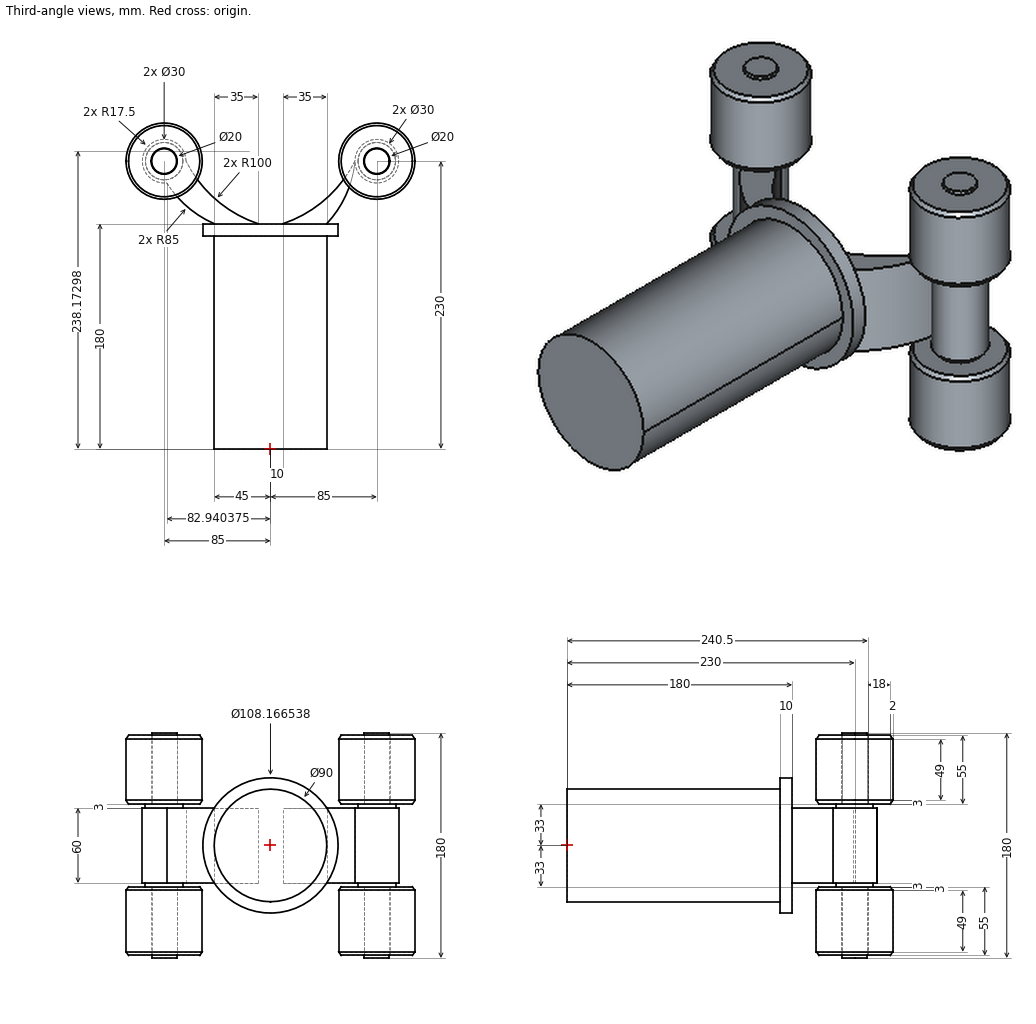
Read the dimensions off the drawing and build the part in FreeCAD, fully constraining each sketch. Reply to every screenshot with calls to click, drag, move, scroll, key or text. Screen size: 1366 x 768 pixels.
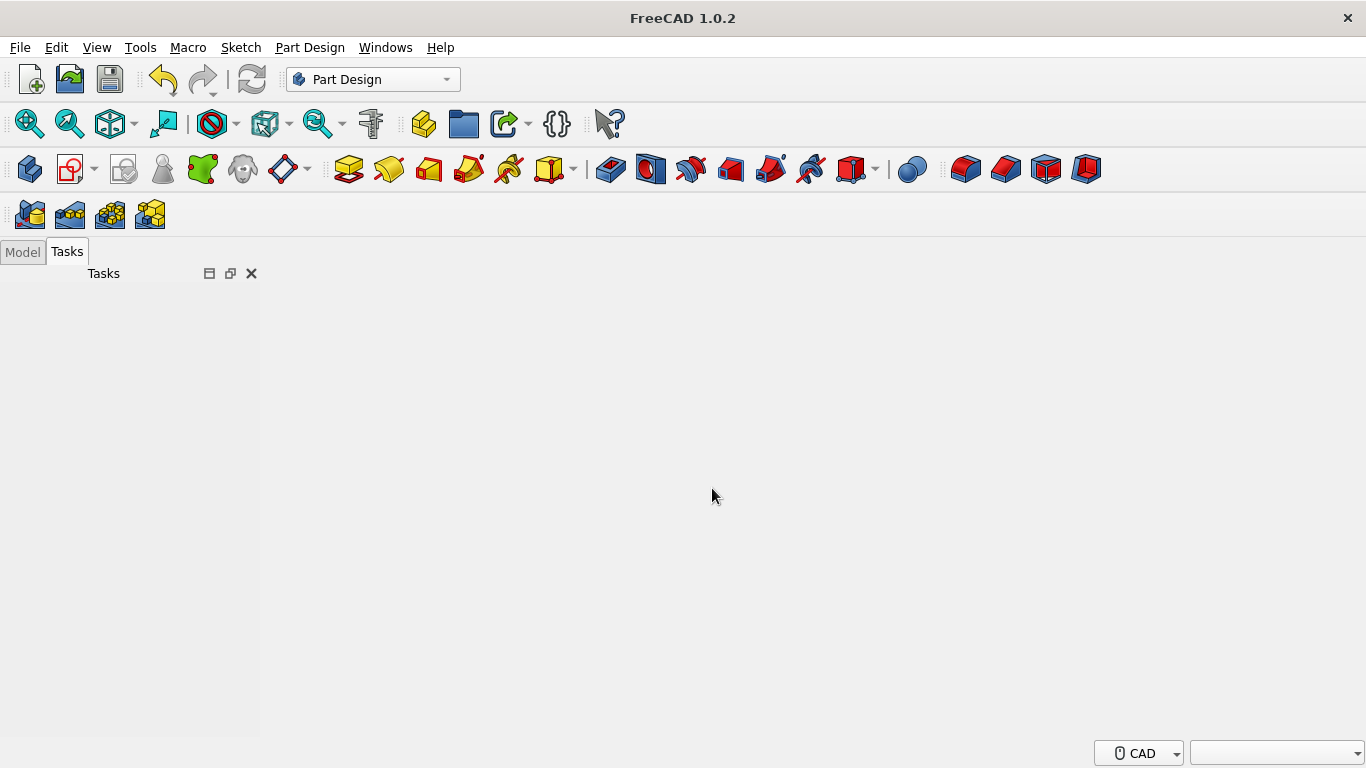
click(30, 80)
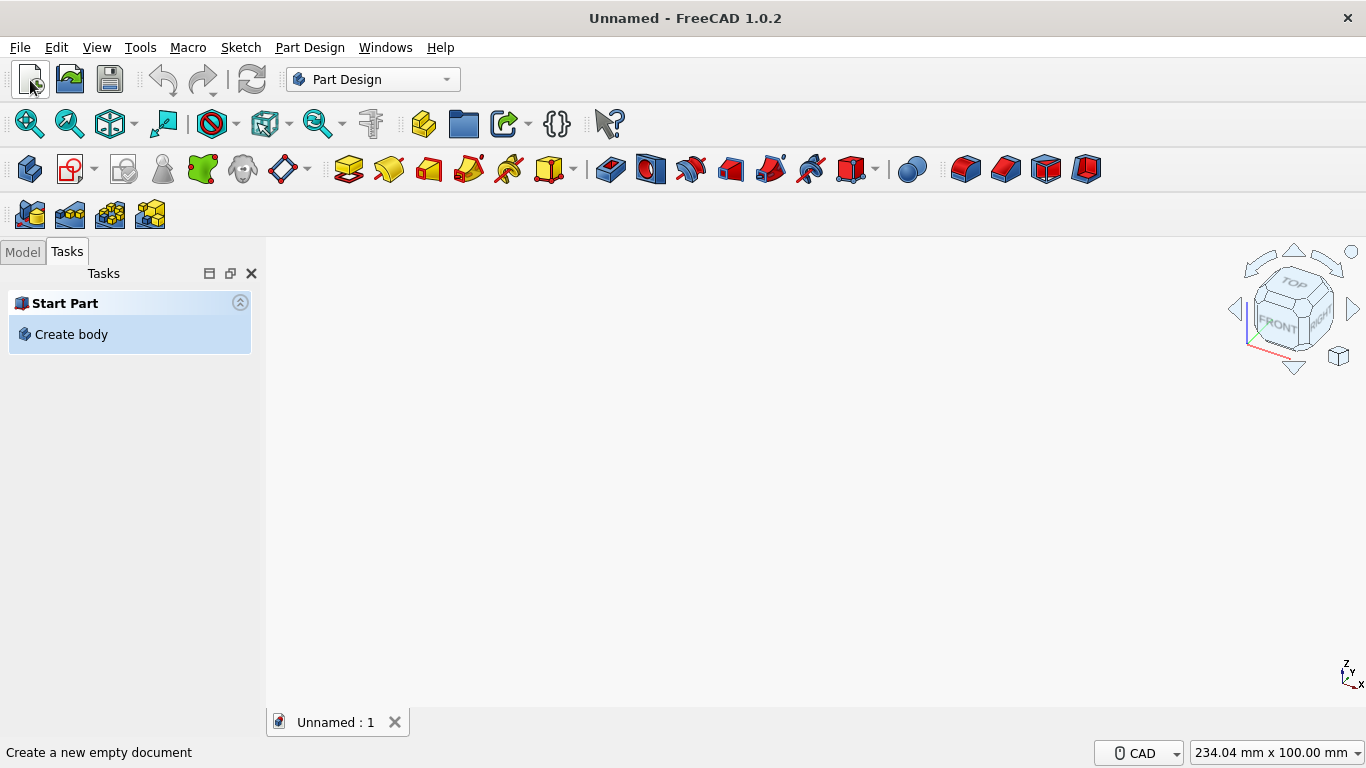
click(70, 170)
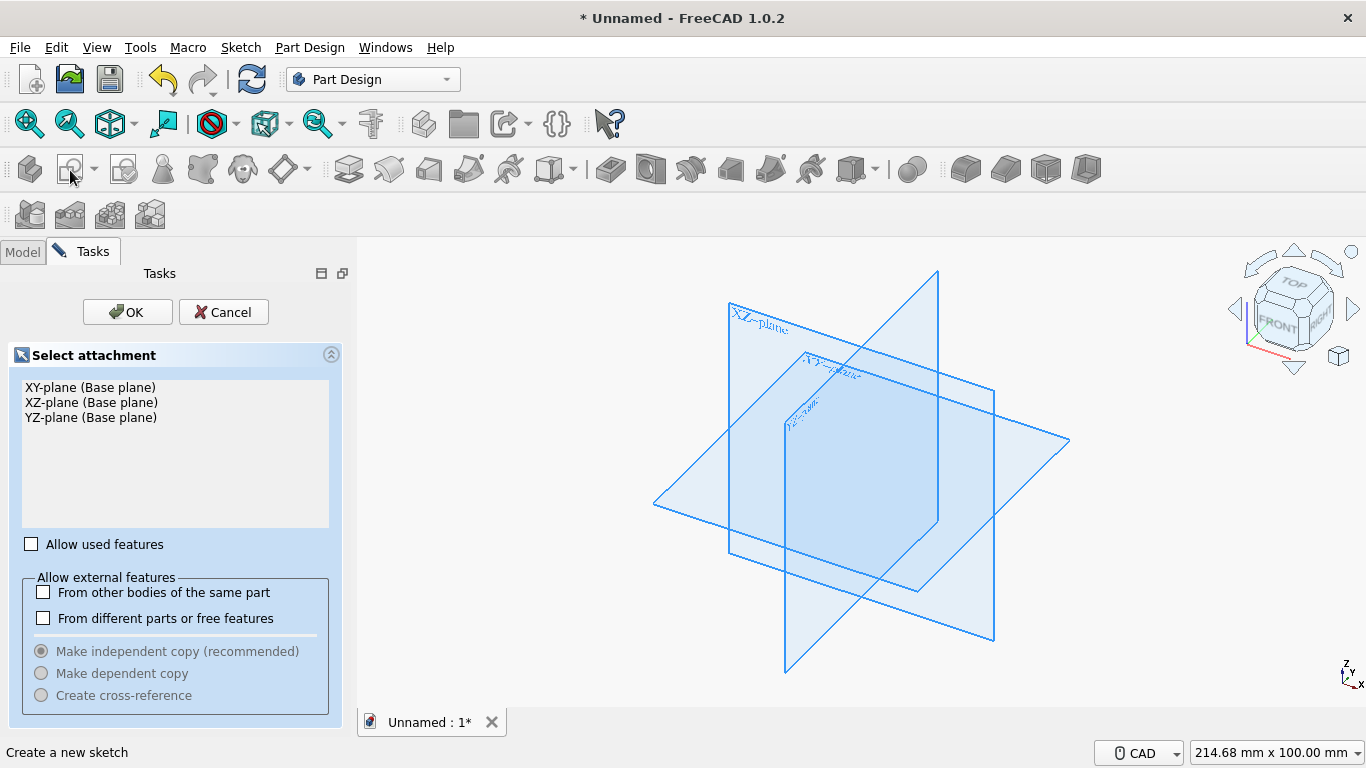
click(82, 402)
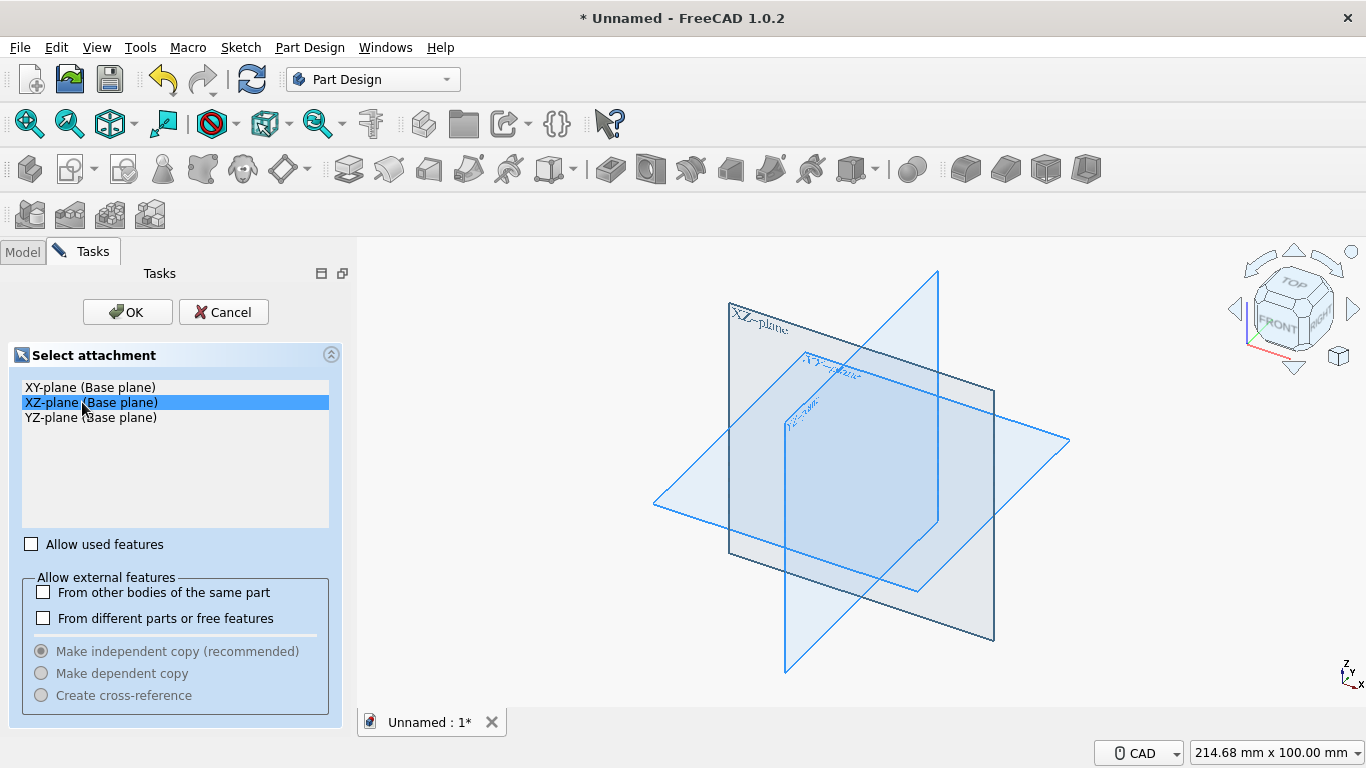
click(128, 312)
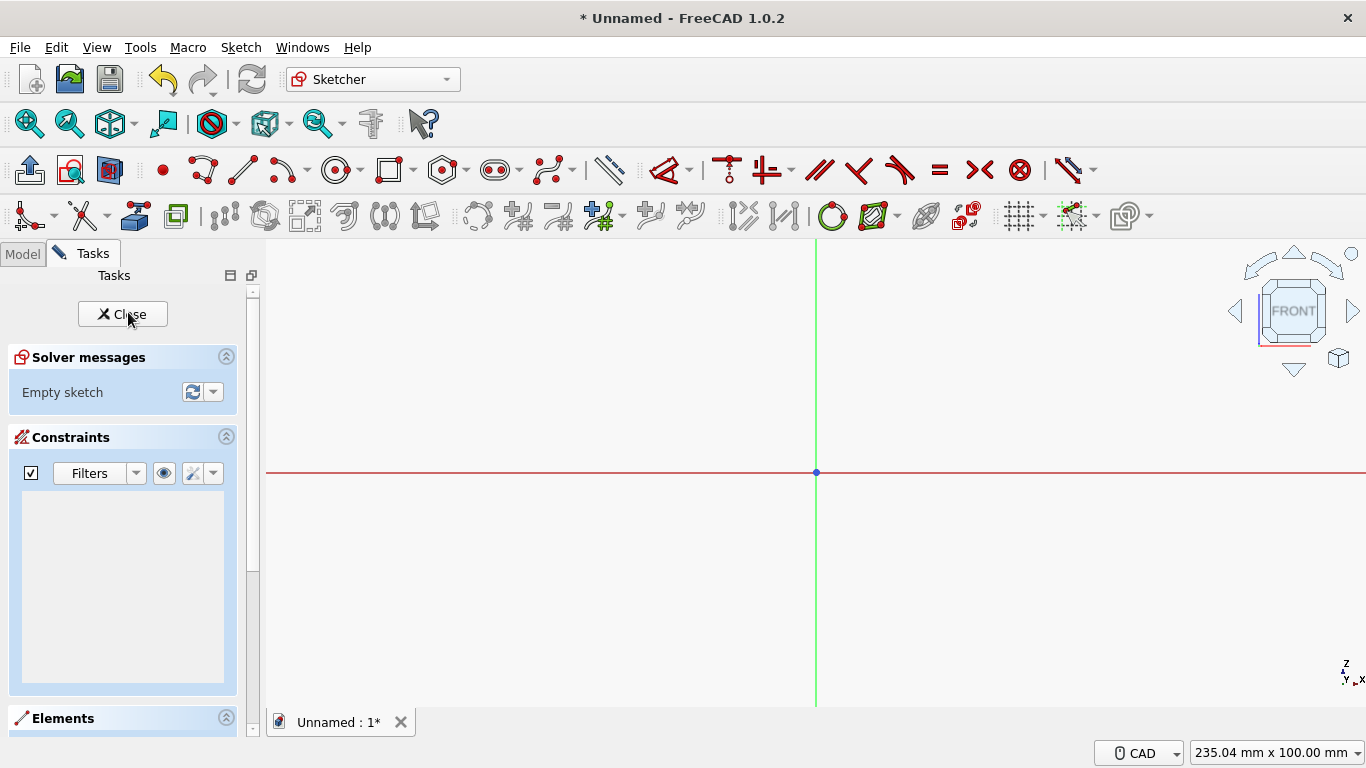
scroll(608, 473, down, 2)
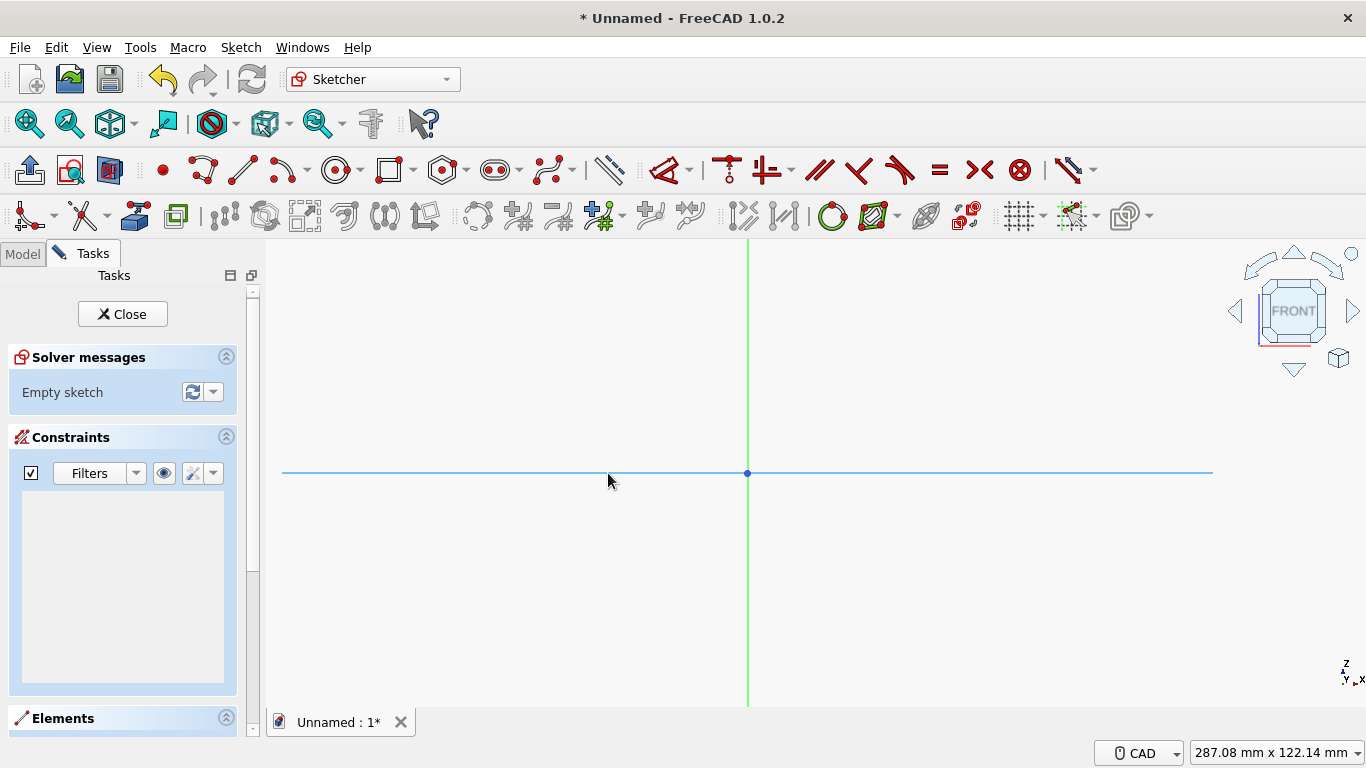
click(336, 170)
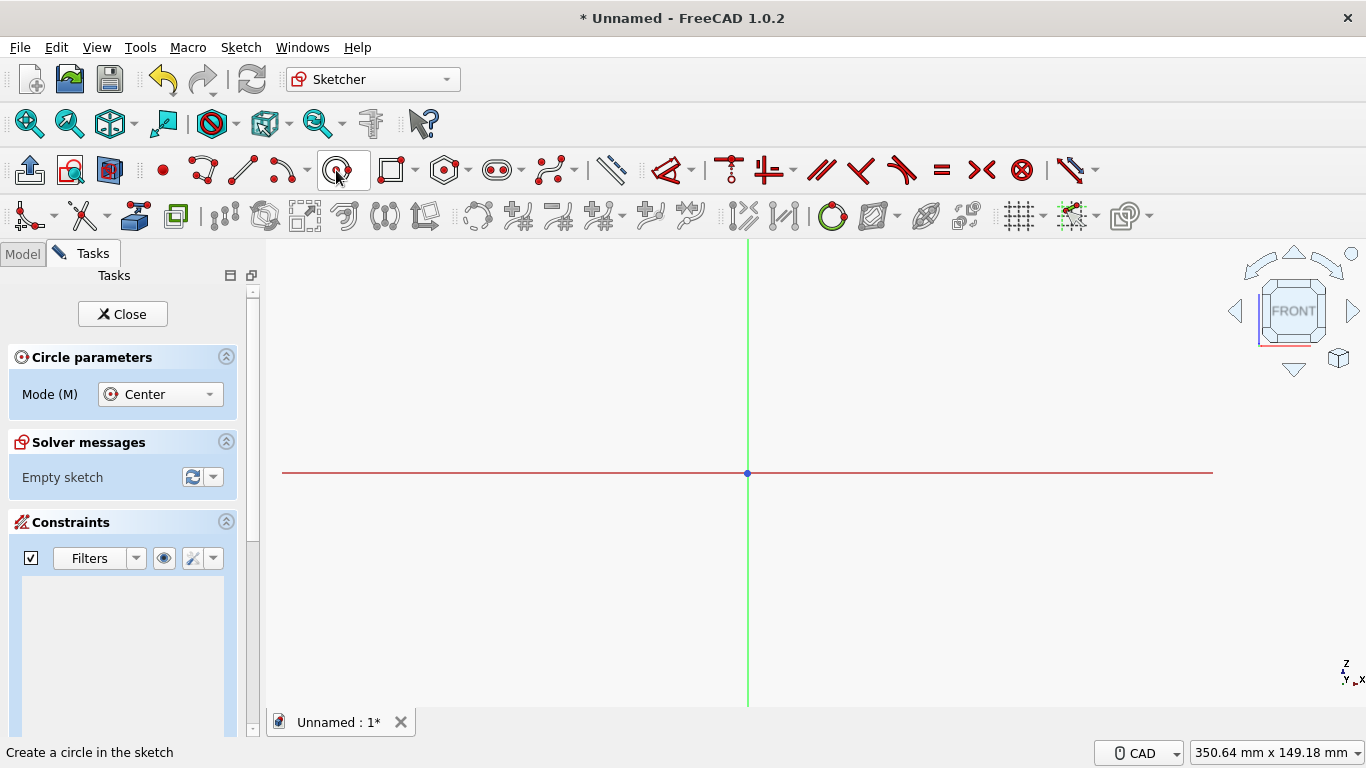
click(748, 473)
click(847, 373)
key(Escape)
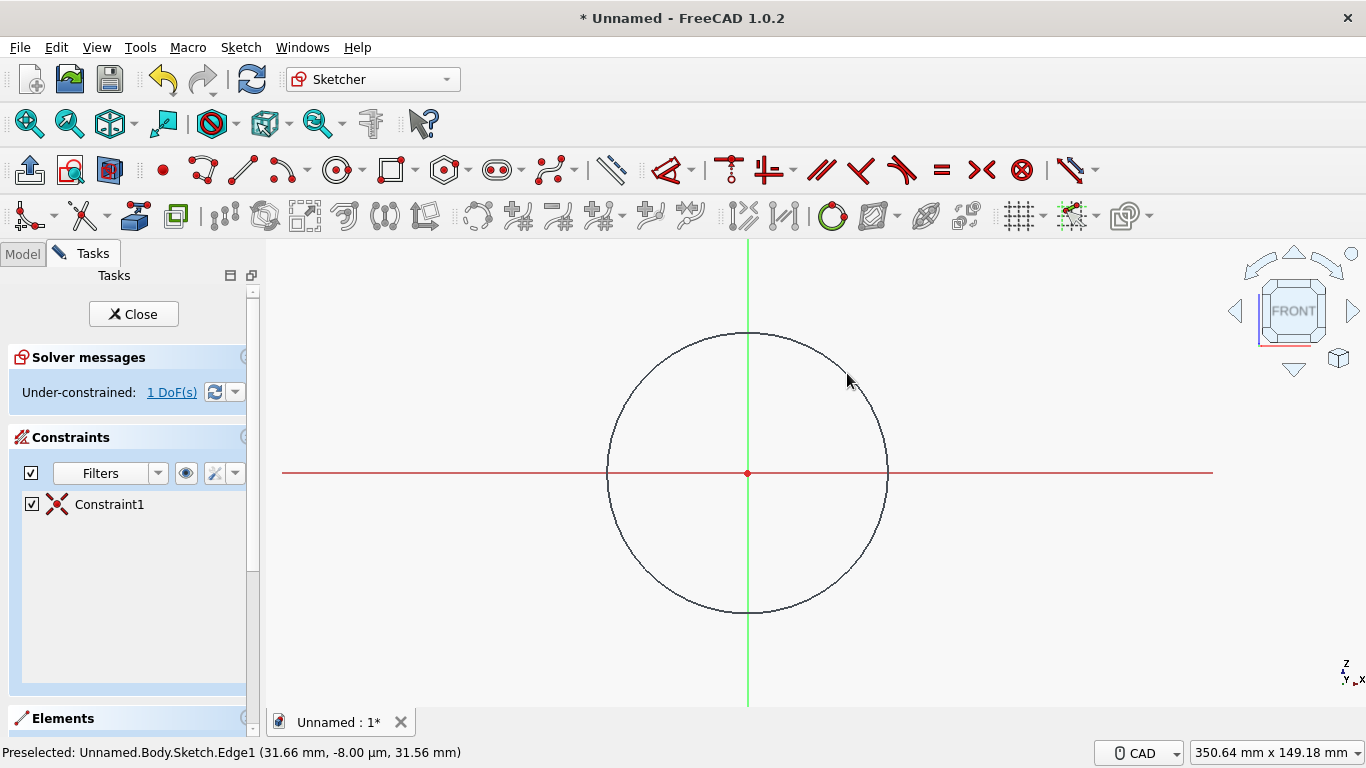
click(666, 170)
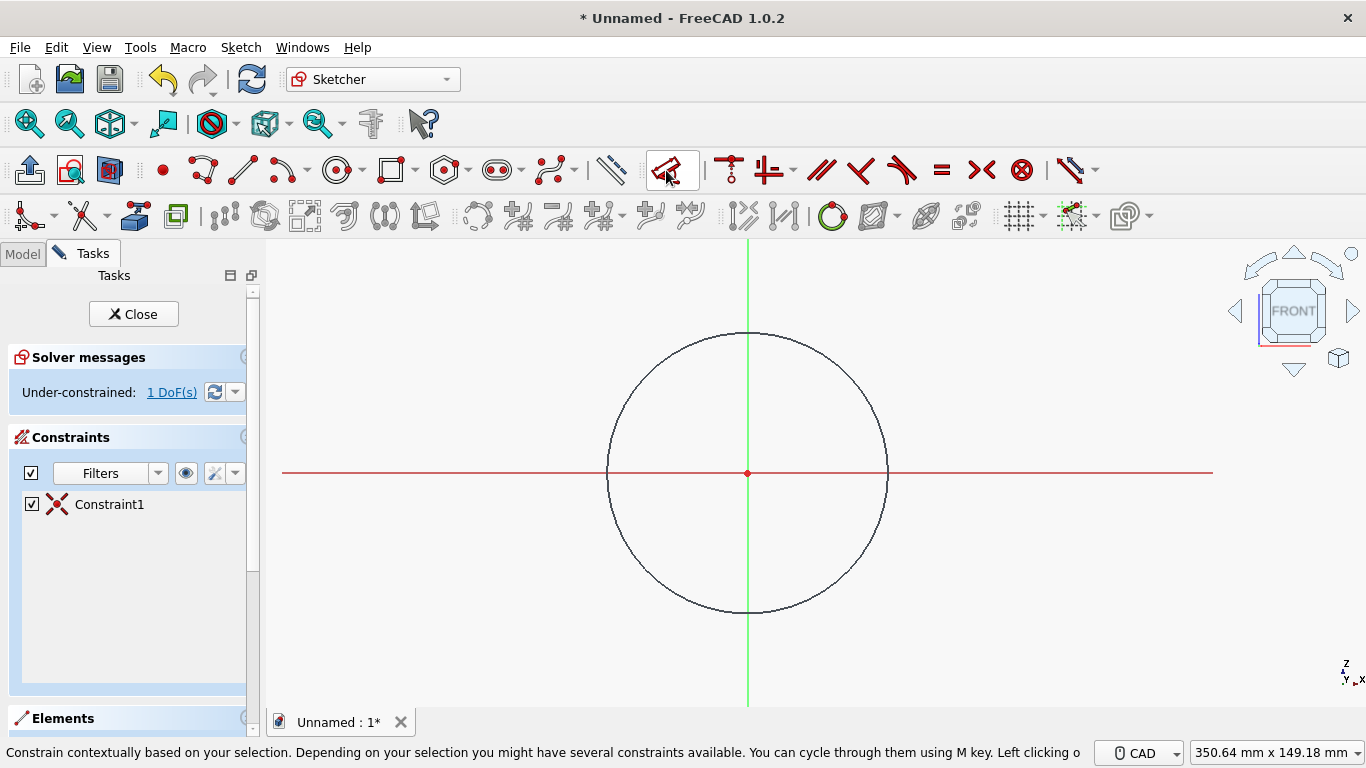
click(847, 374)
click(870, 351)